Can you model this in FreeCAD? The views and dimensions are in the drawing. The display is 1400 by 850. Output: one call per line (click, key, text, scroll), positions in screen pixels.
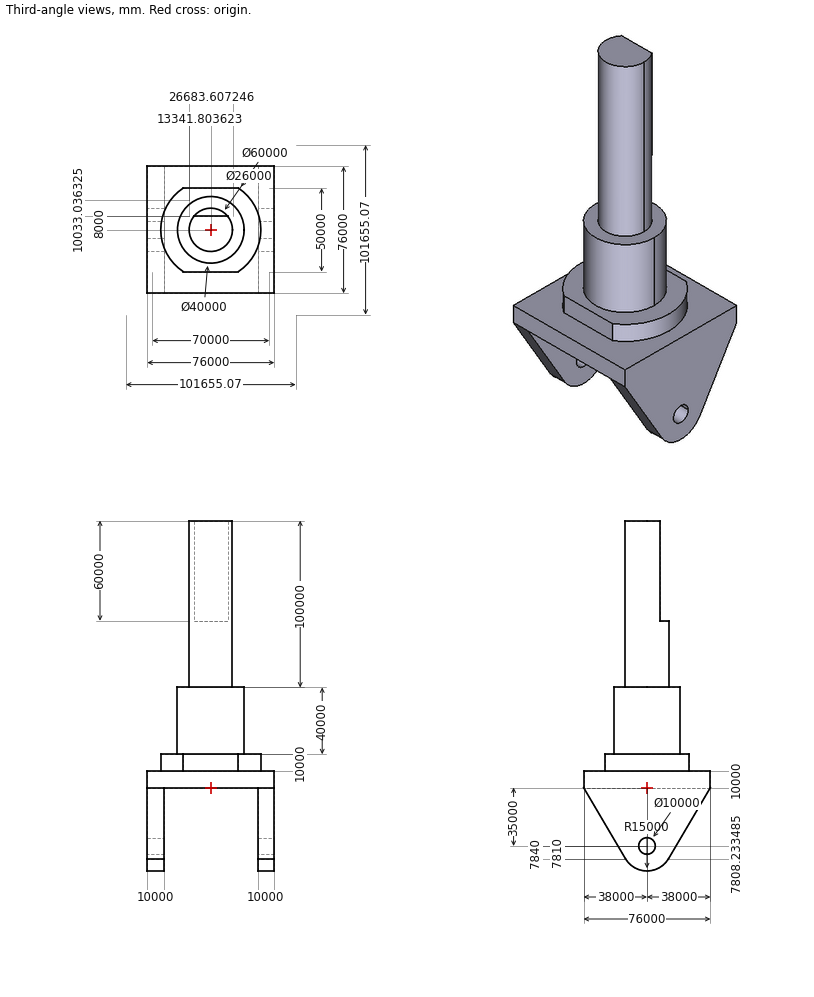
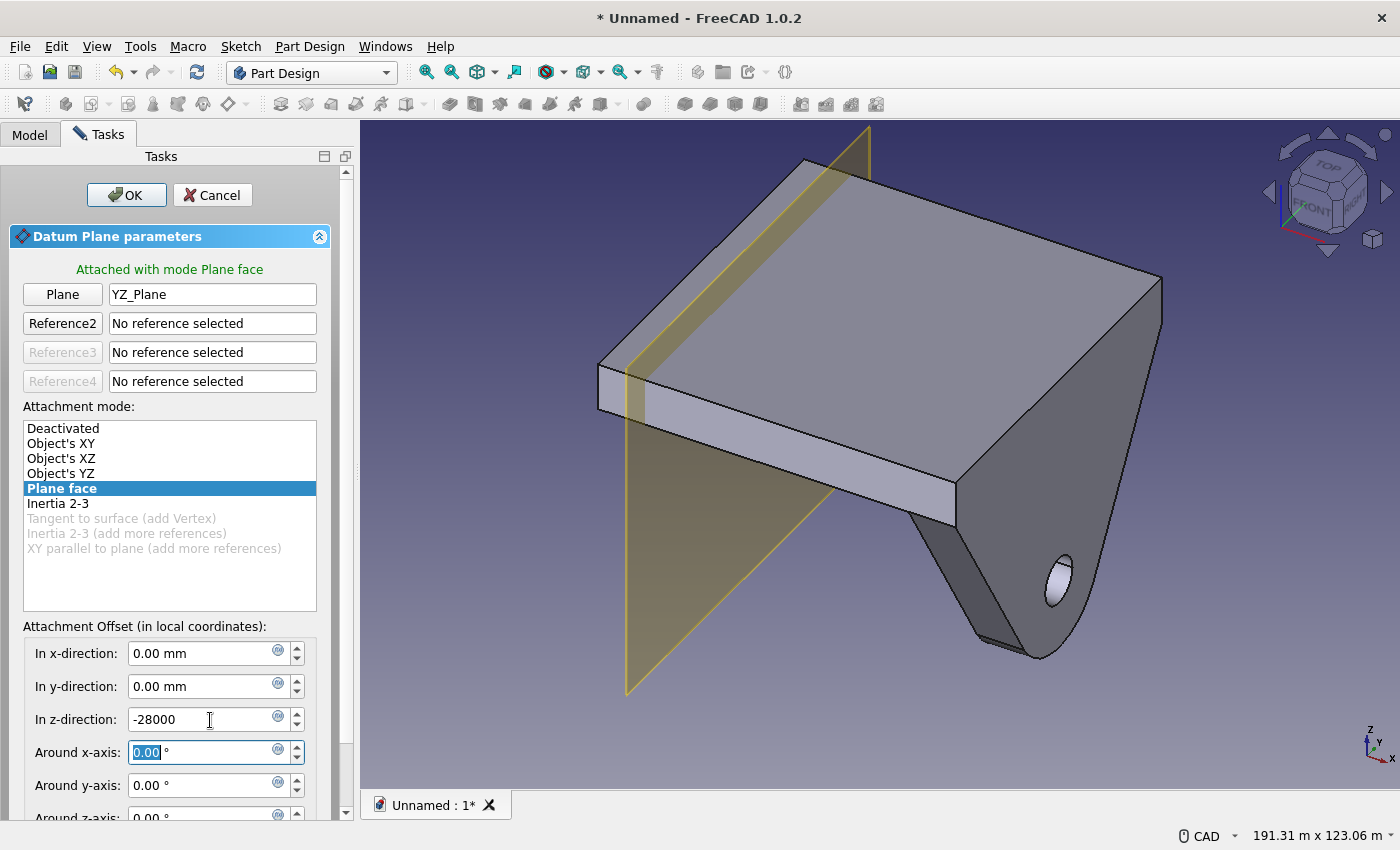
click(127, 195)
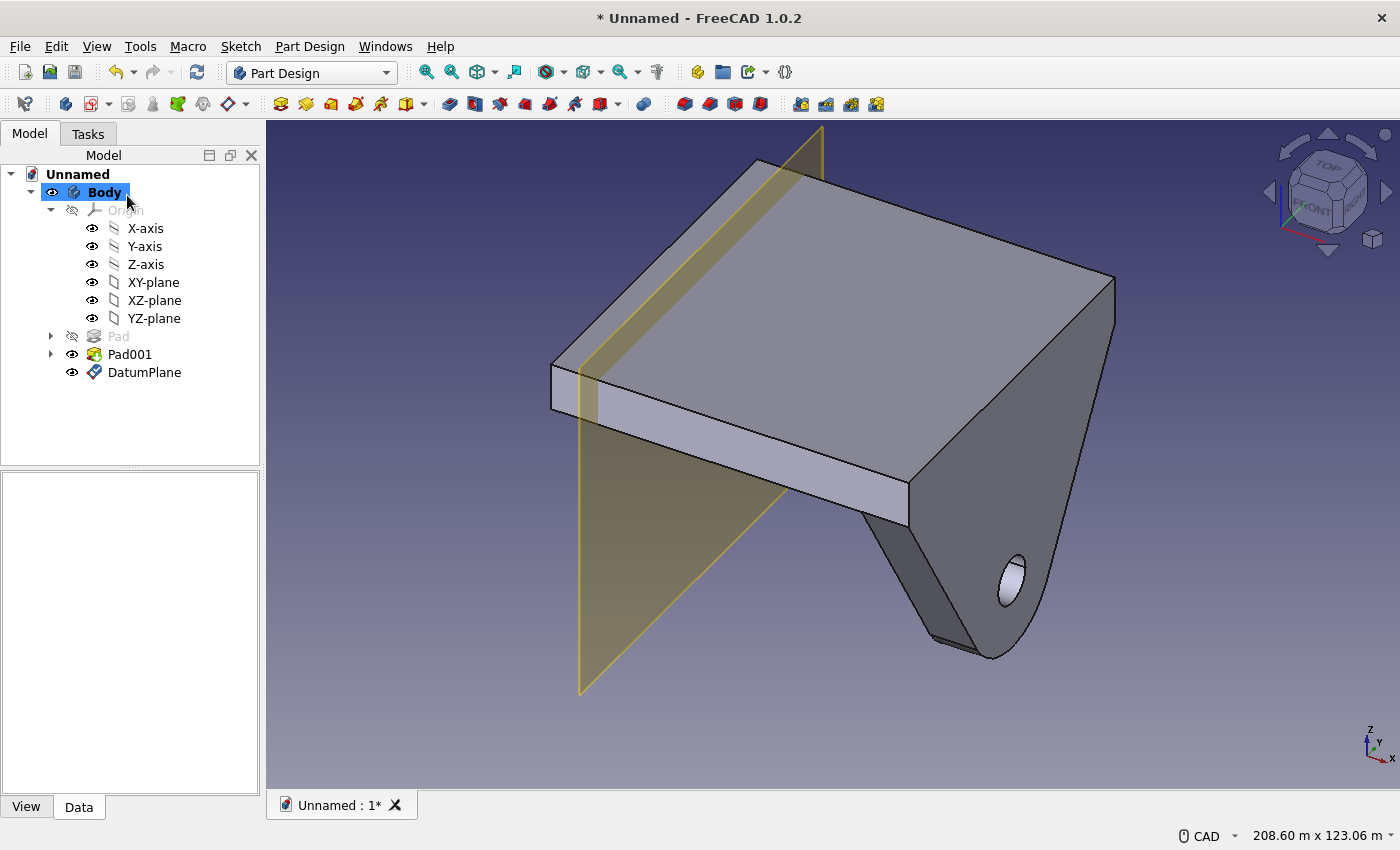
click(117, 372)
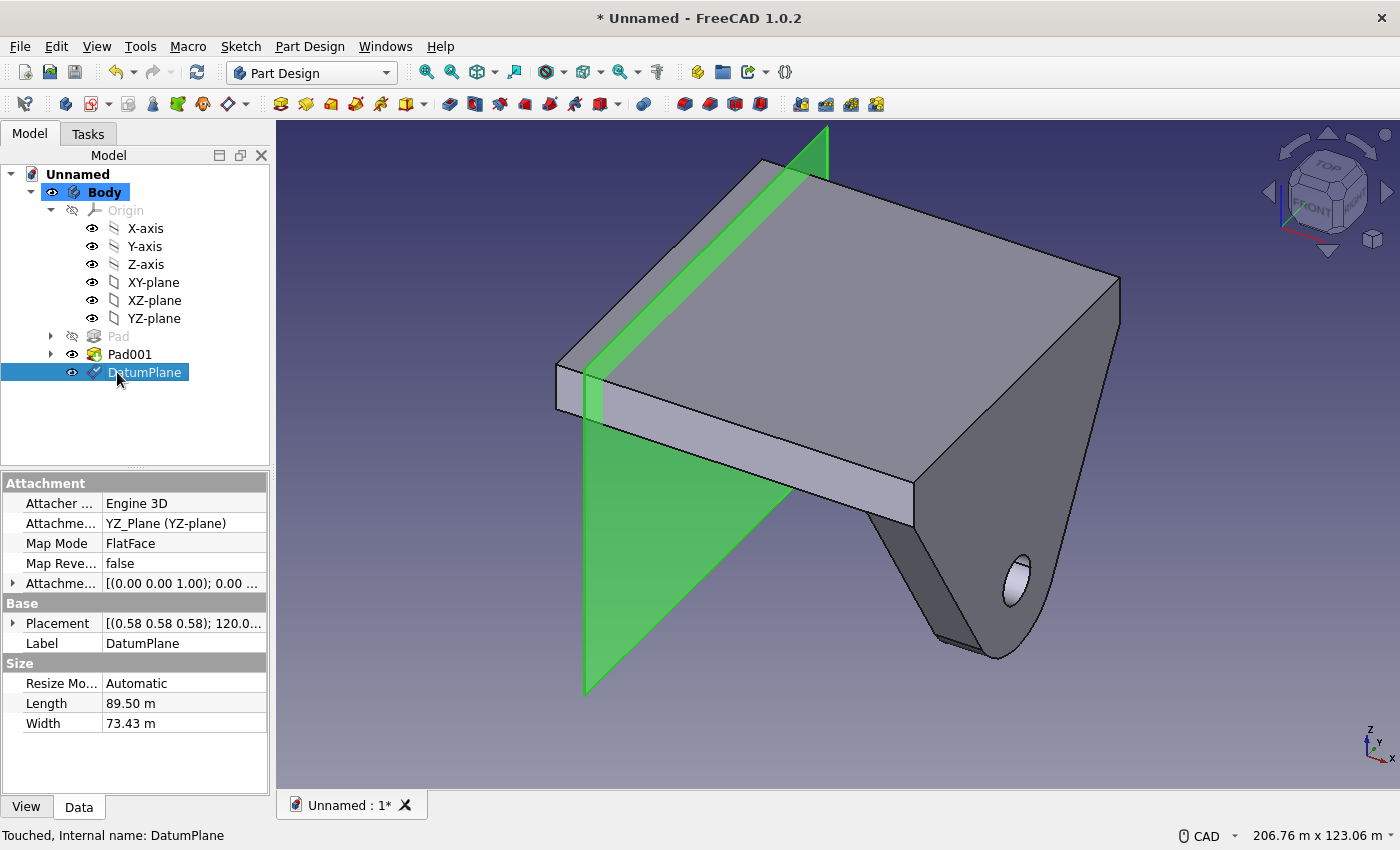
click(90, 104)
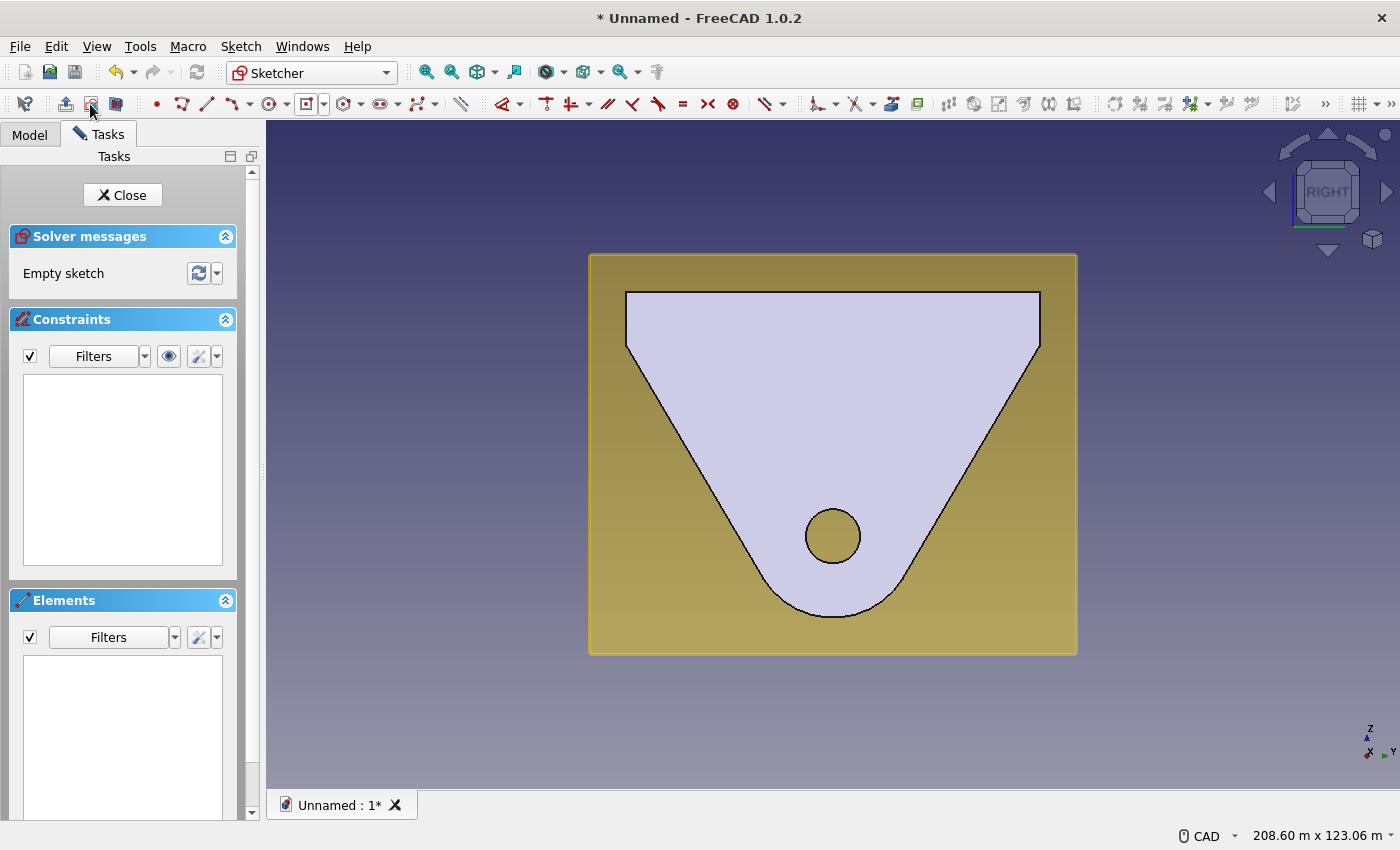
click(116, 104)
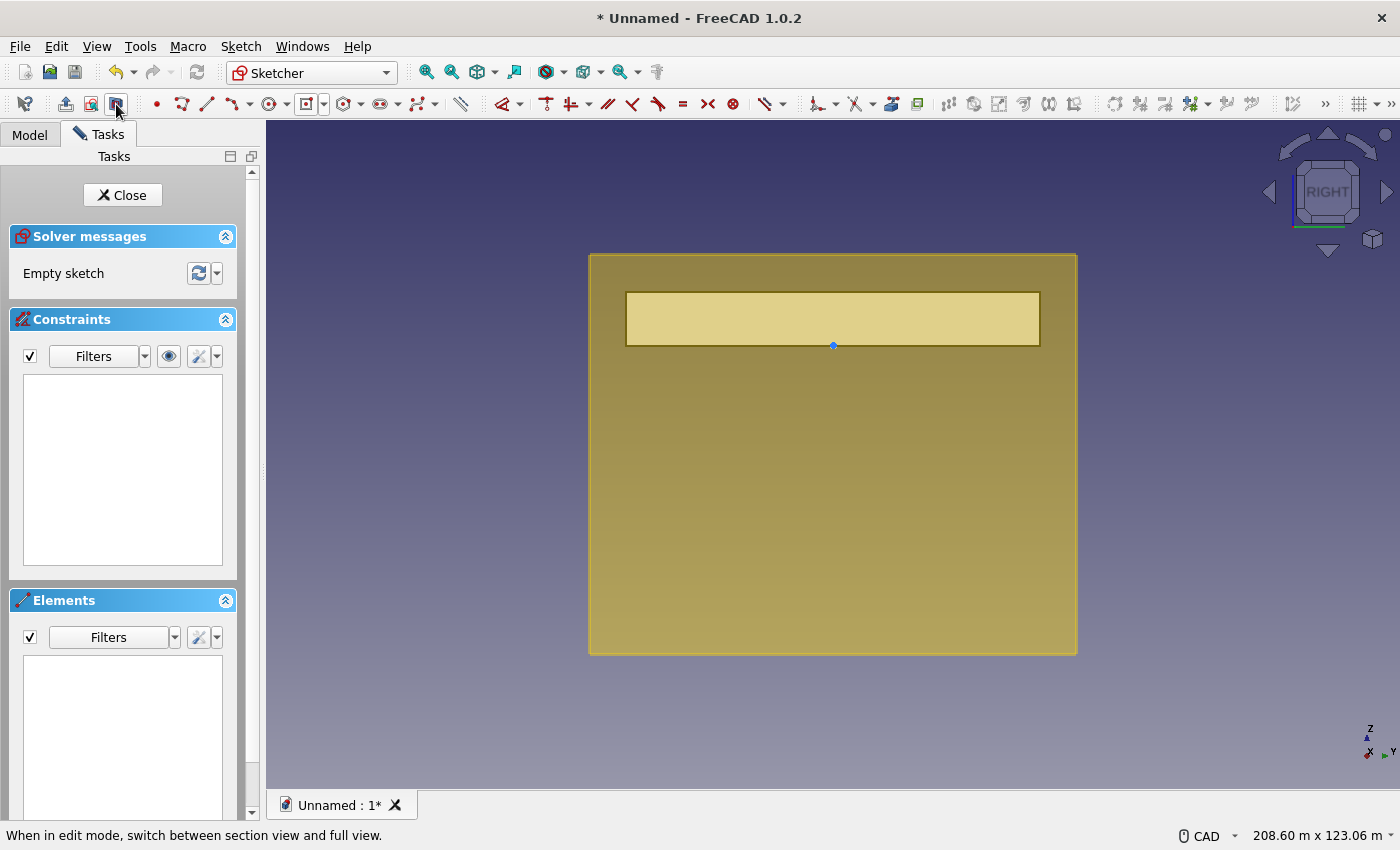
scroll(972, 537, up, 2)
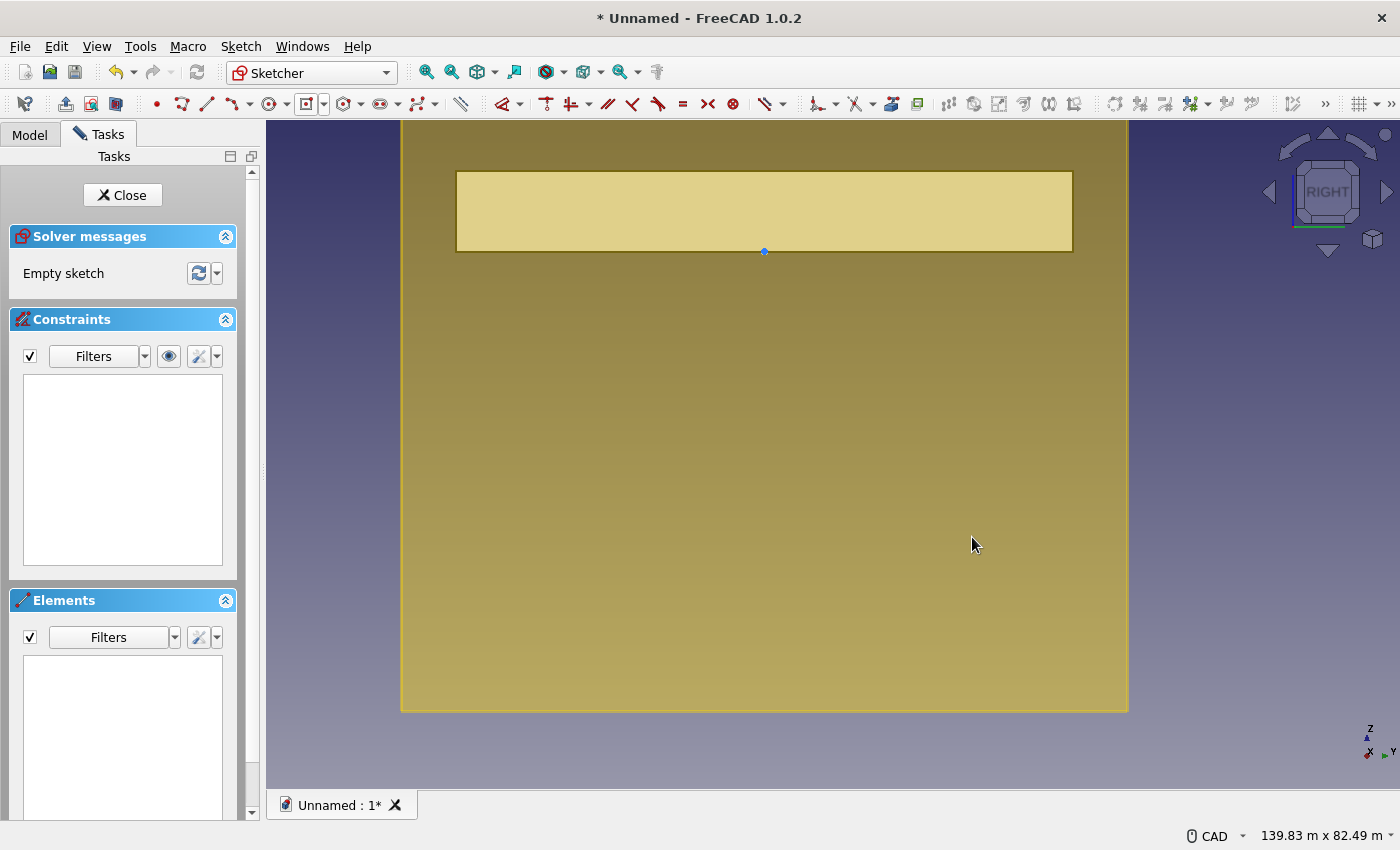
click(182, 104)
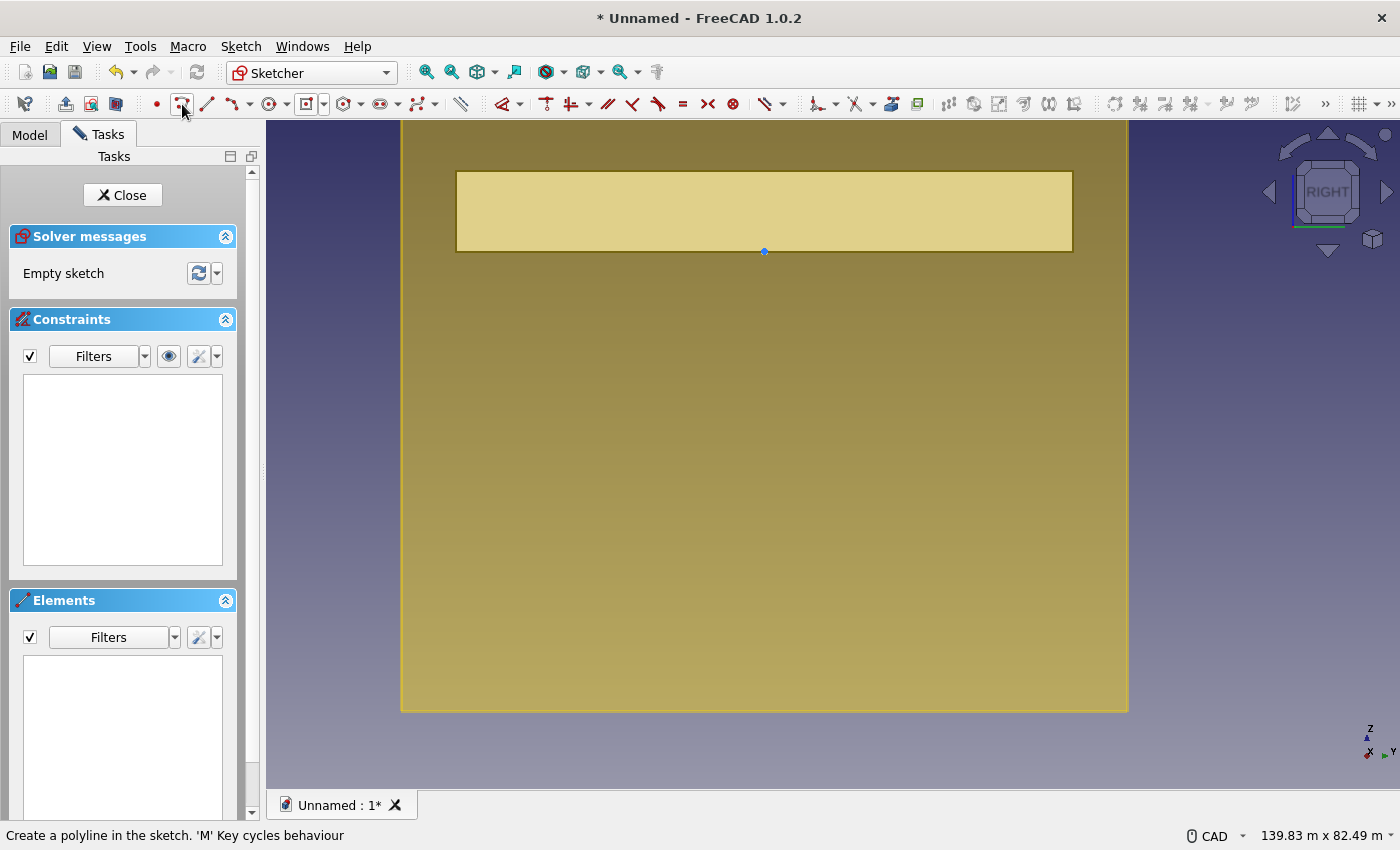
click(661, 599)
click(456, 252)
click(1073, 261)
click(868, 599)
right_click(868, 599)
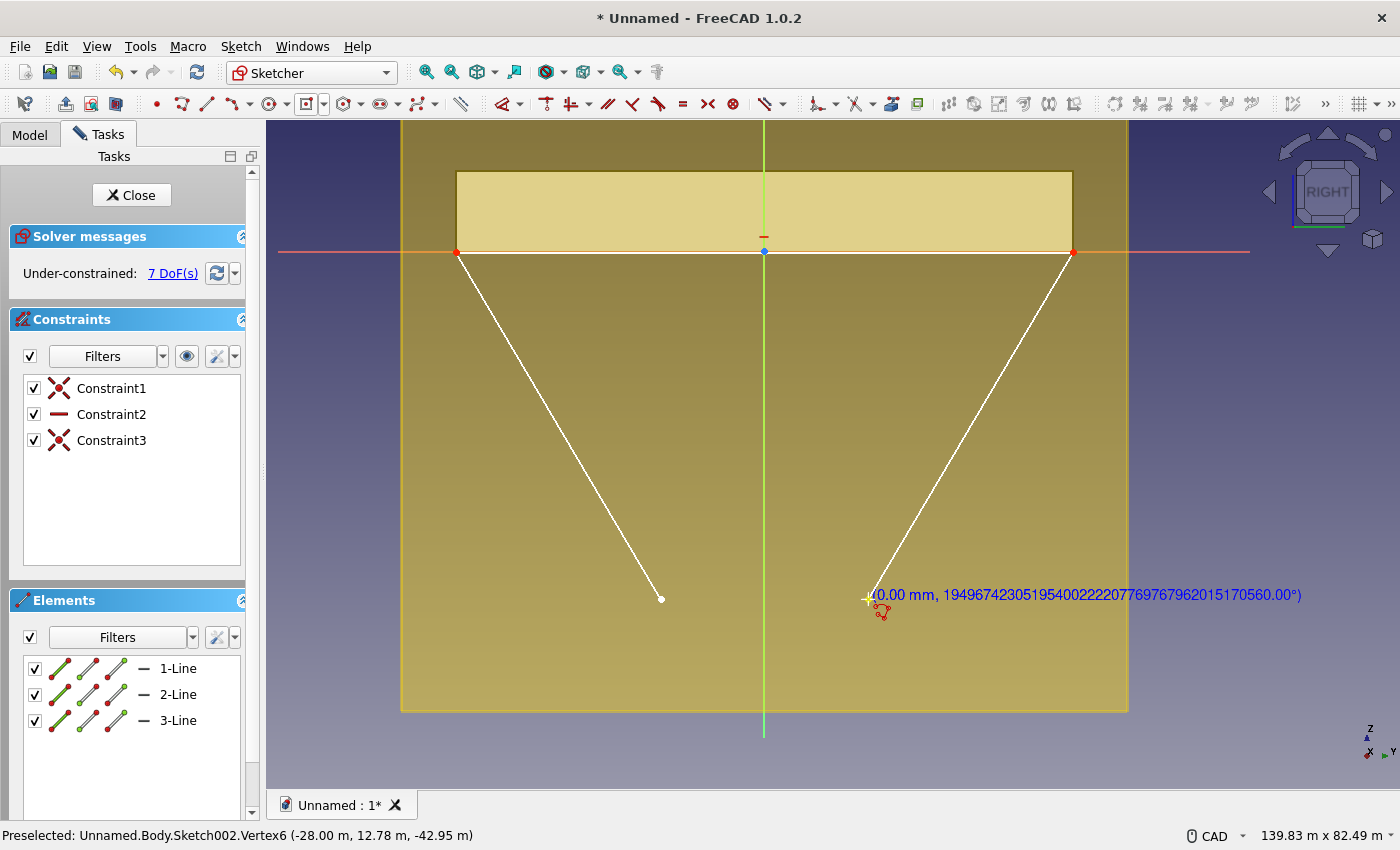
click(232, 104)